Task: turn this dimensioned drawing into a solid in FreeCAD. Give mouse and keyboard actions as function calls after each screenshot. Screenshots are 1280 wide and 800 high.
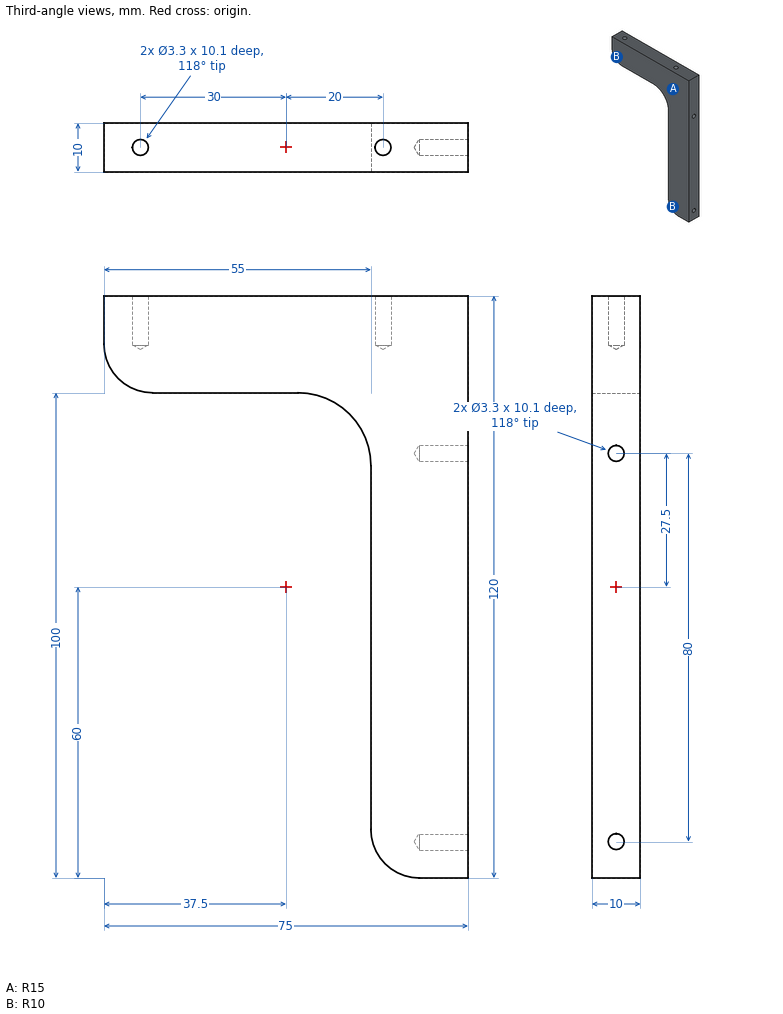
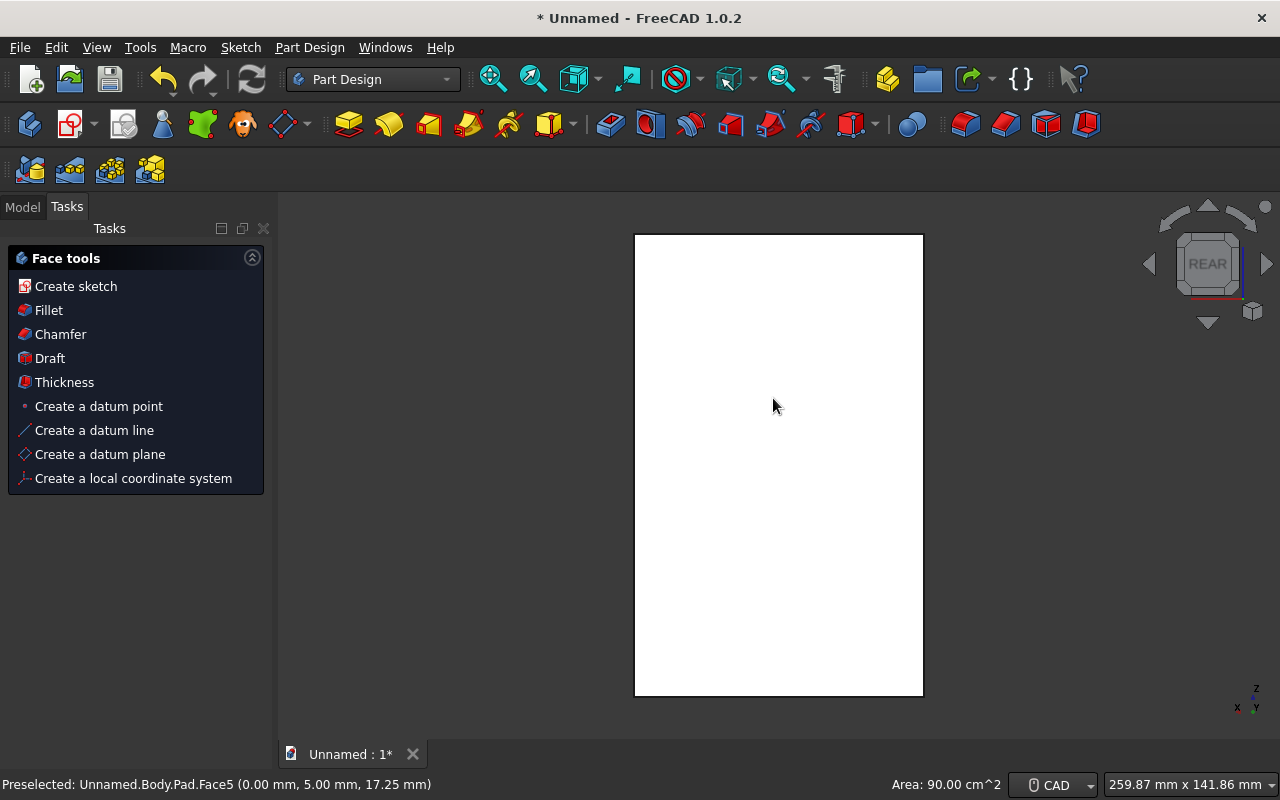
click(70, 124)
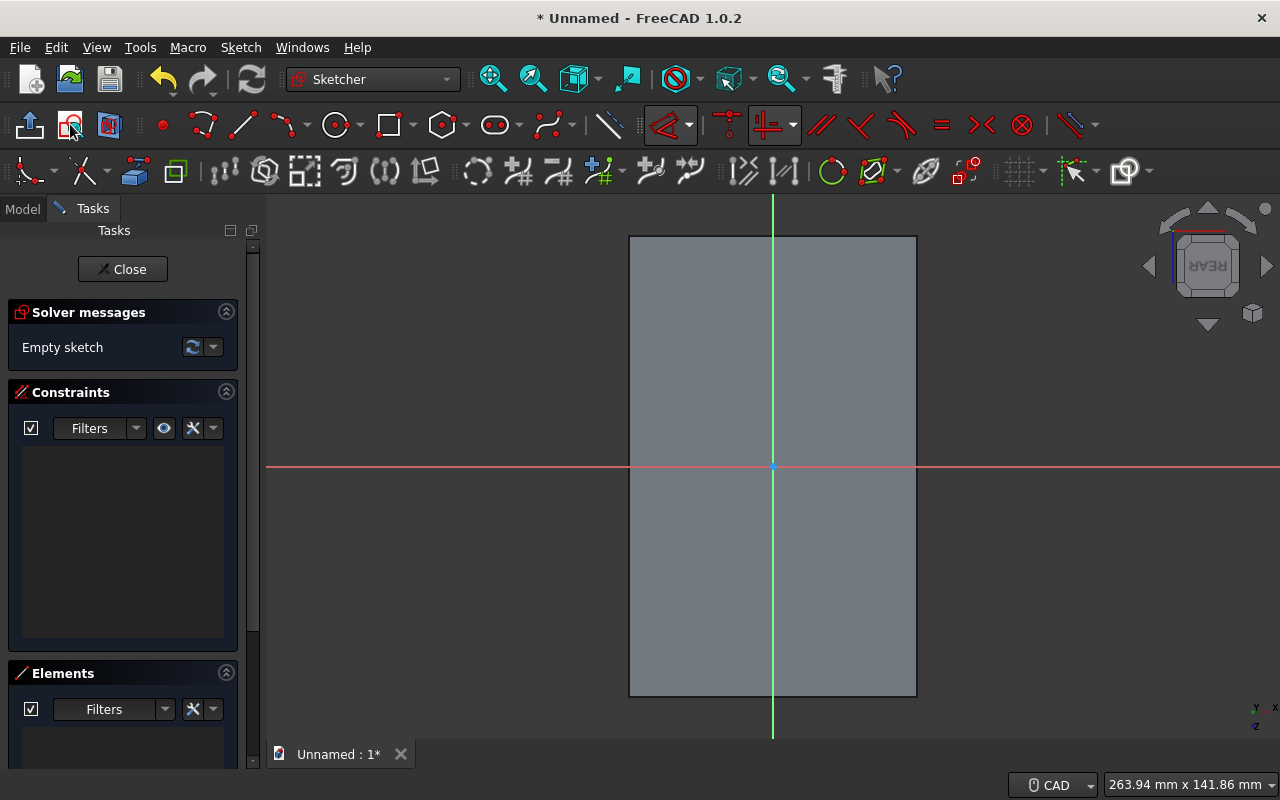
scroll(569, 640, down, 1)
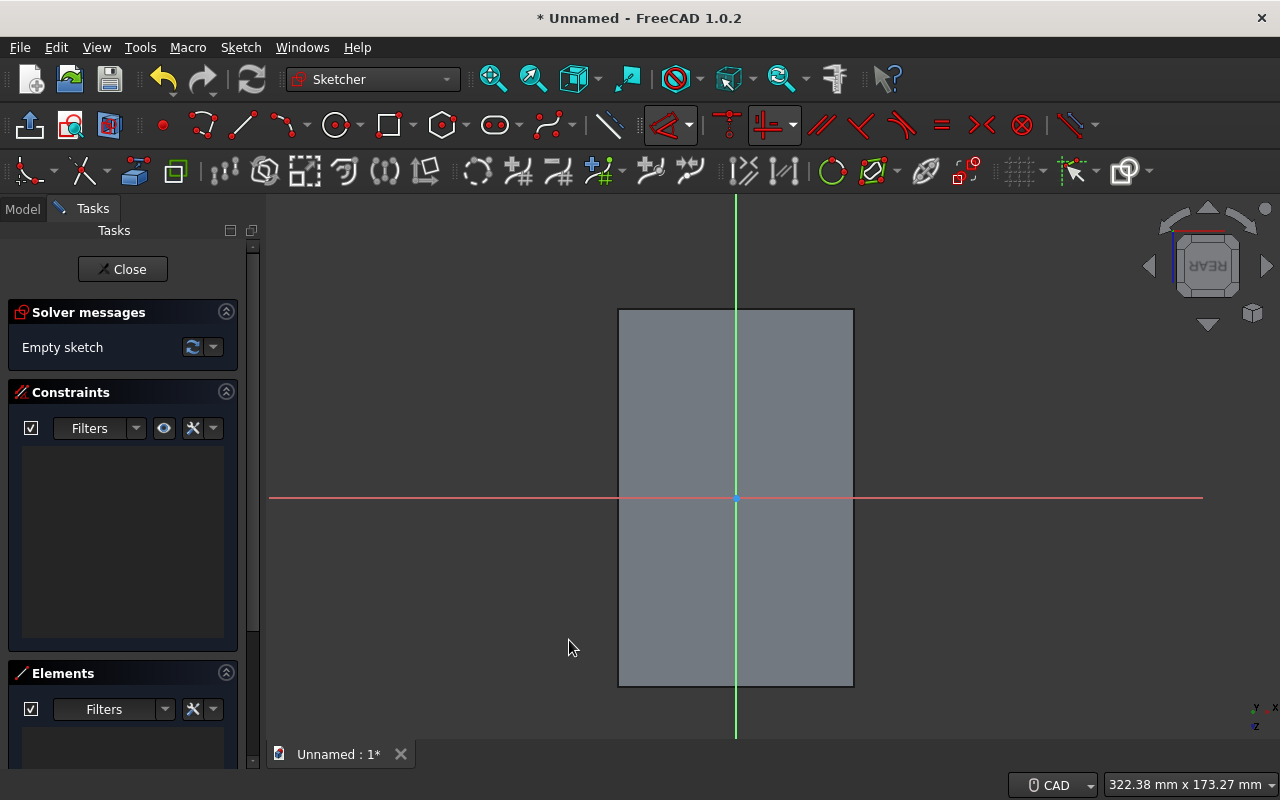
click(390, 126)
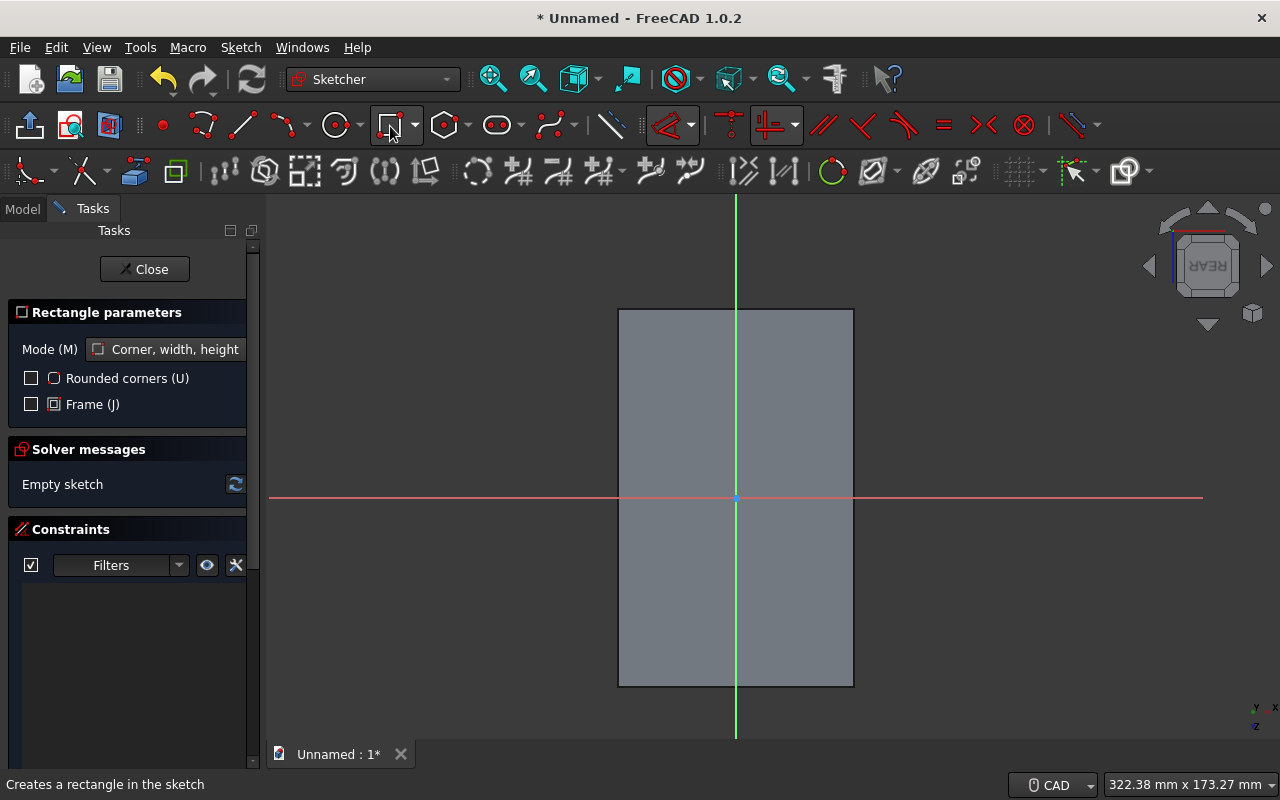
click(618, 309)
click(791, 624)
key(Escape)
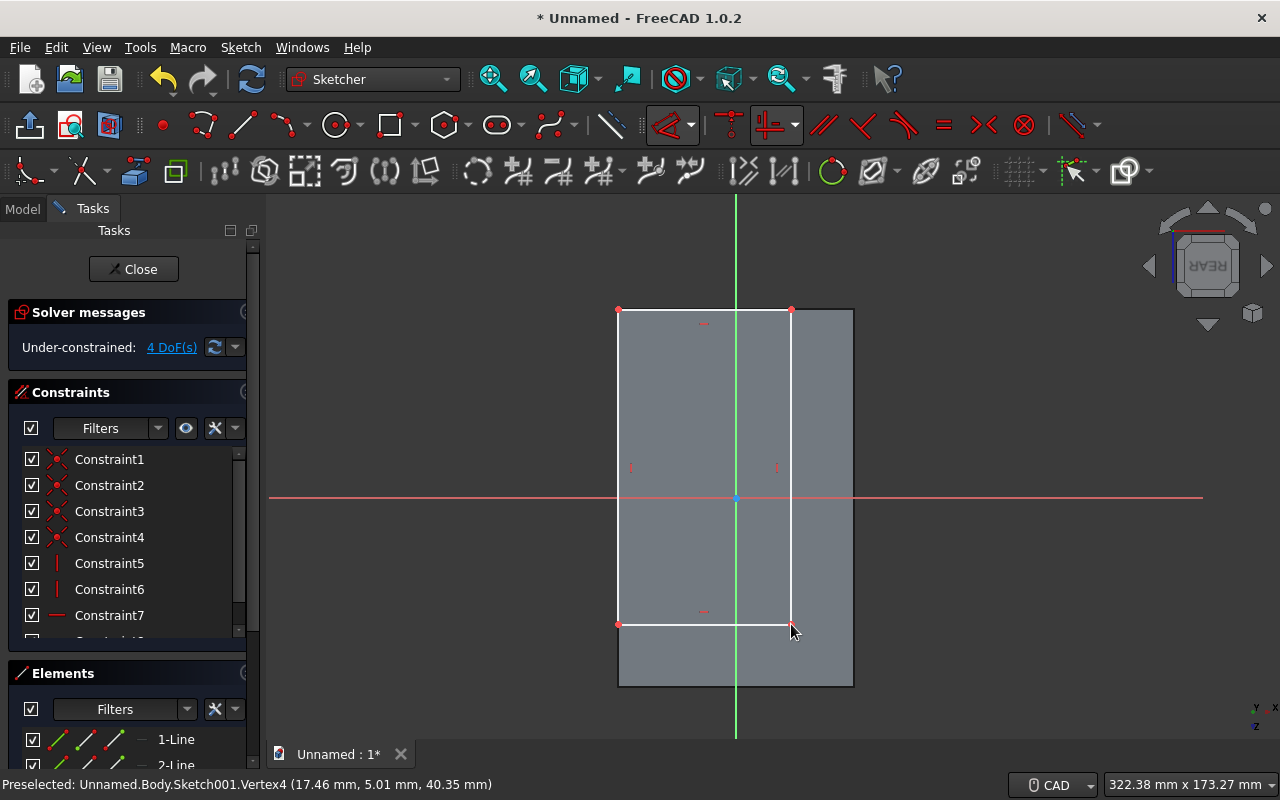
key(d)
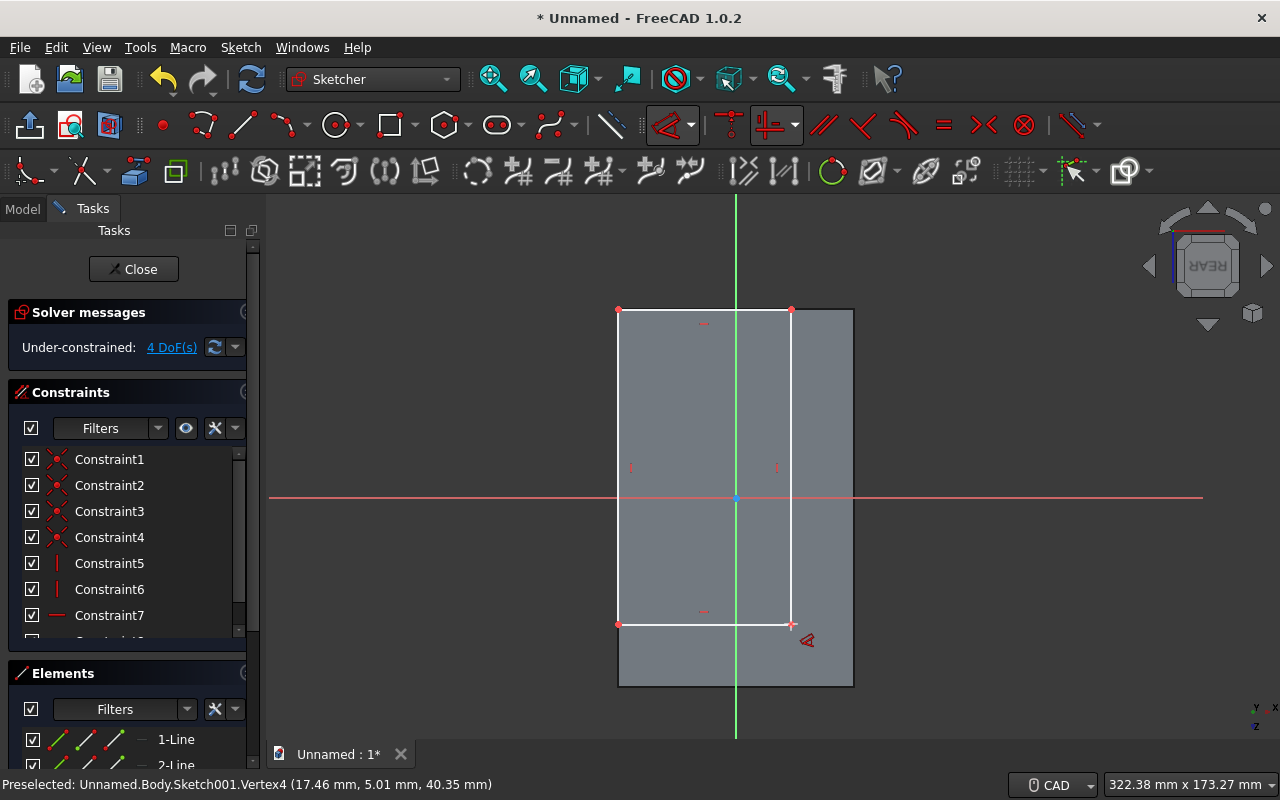
click(670, 625)
click(704, 659)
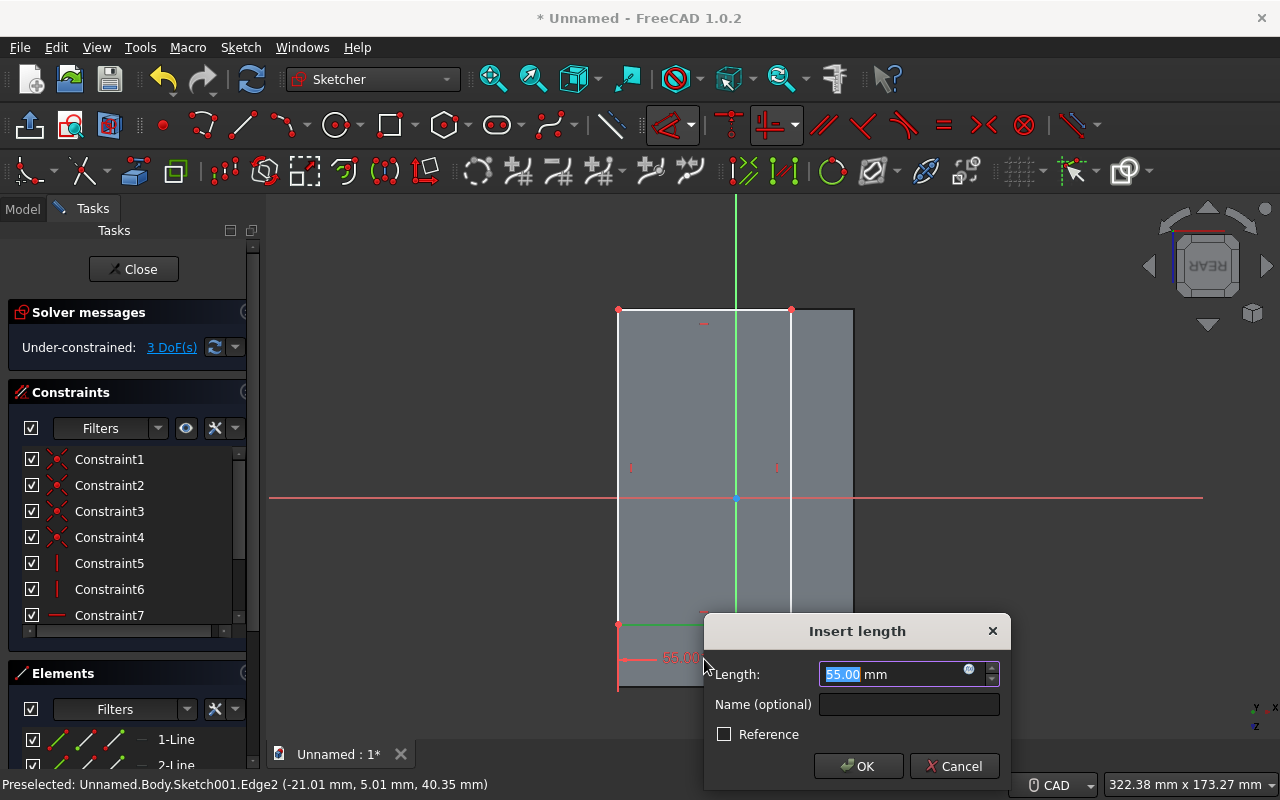
text(55)
key(Return)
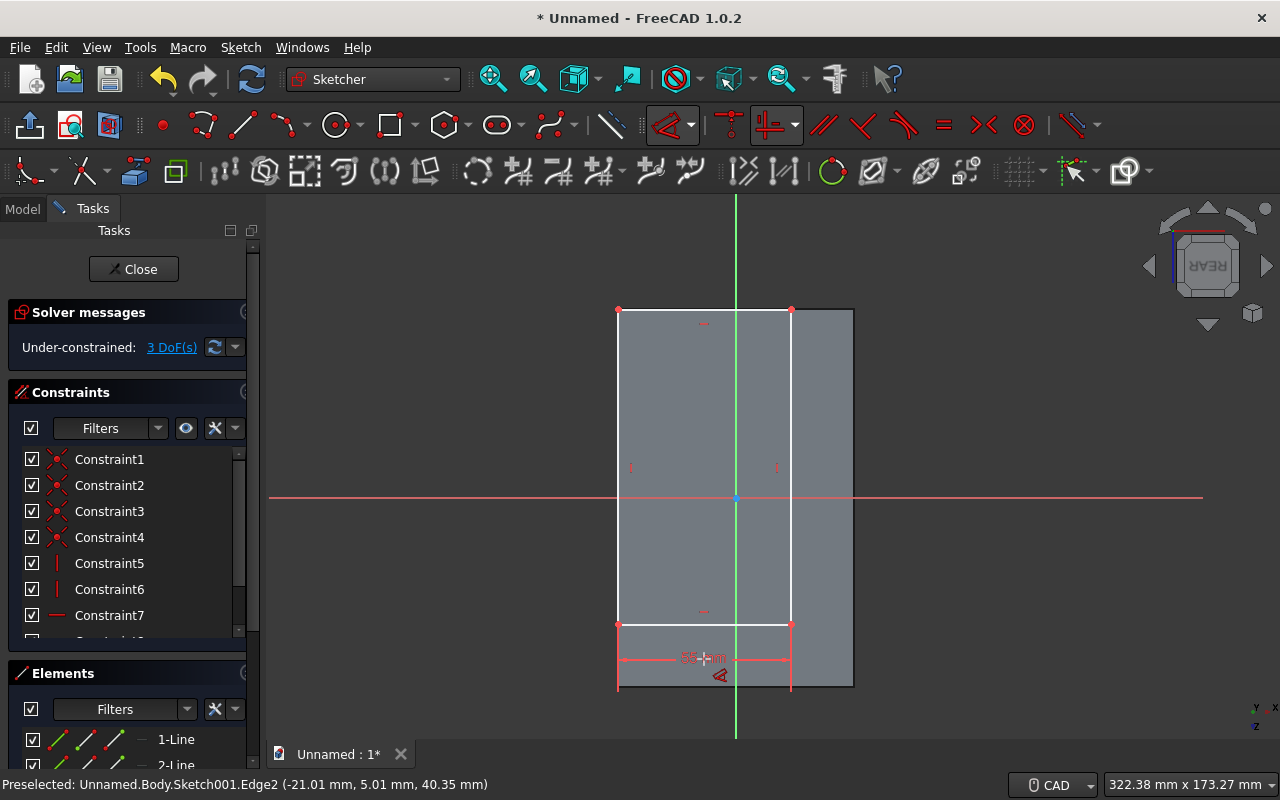
click(618, 404)
click(584, 467)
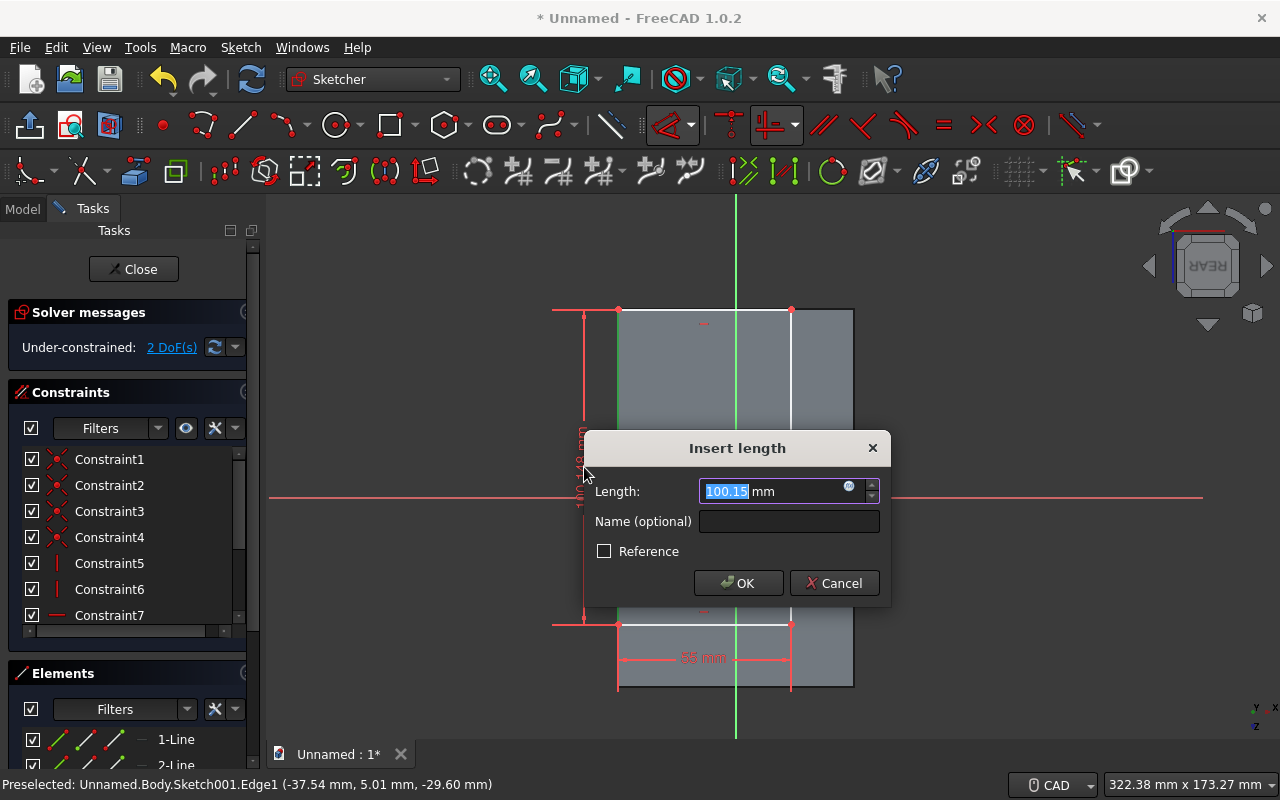
text(100)
key(Return)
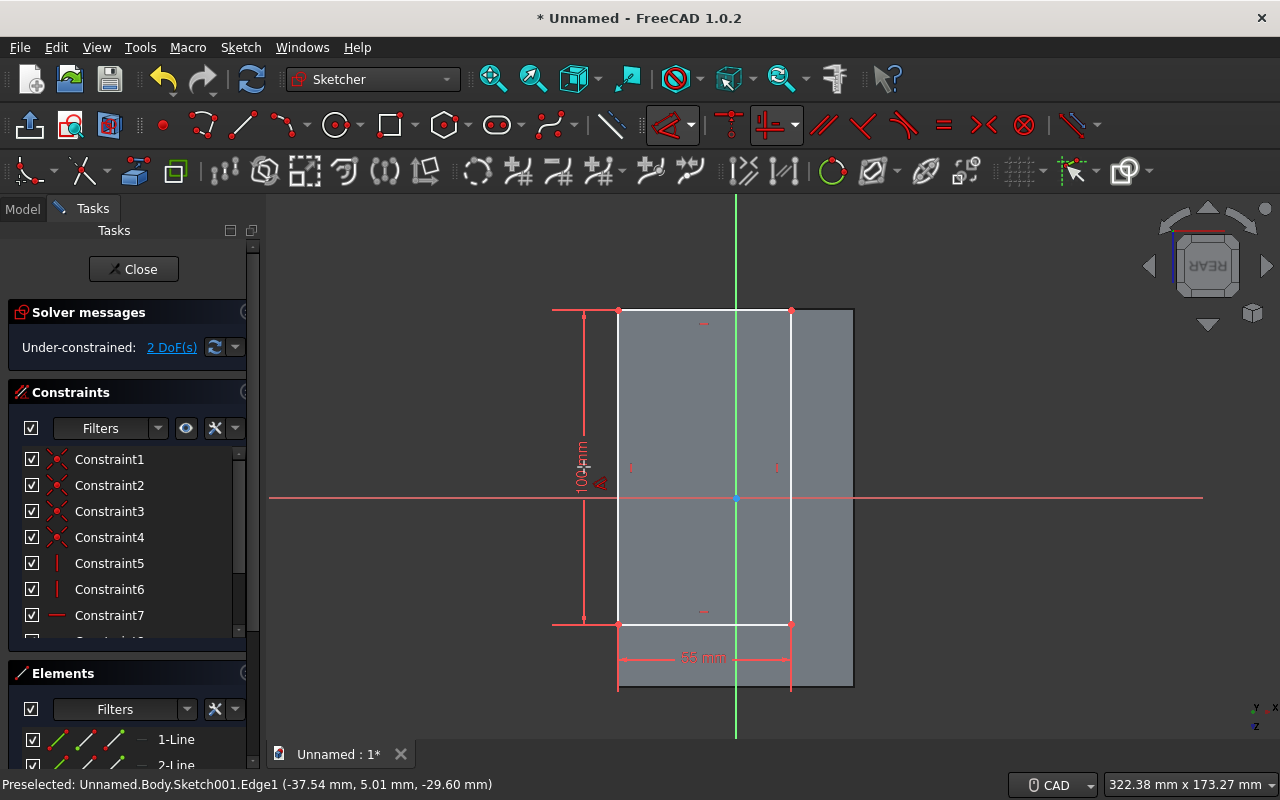
click(618, 310)
click(584, 404)